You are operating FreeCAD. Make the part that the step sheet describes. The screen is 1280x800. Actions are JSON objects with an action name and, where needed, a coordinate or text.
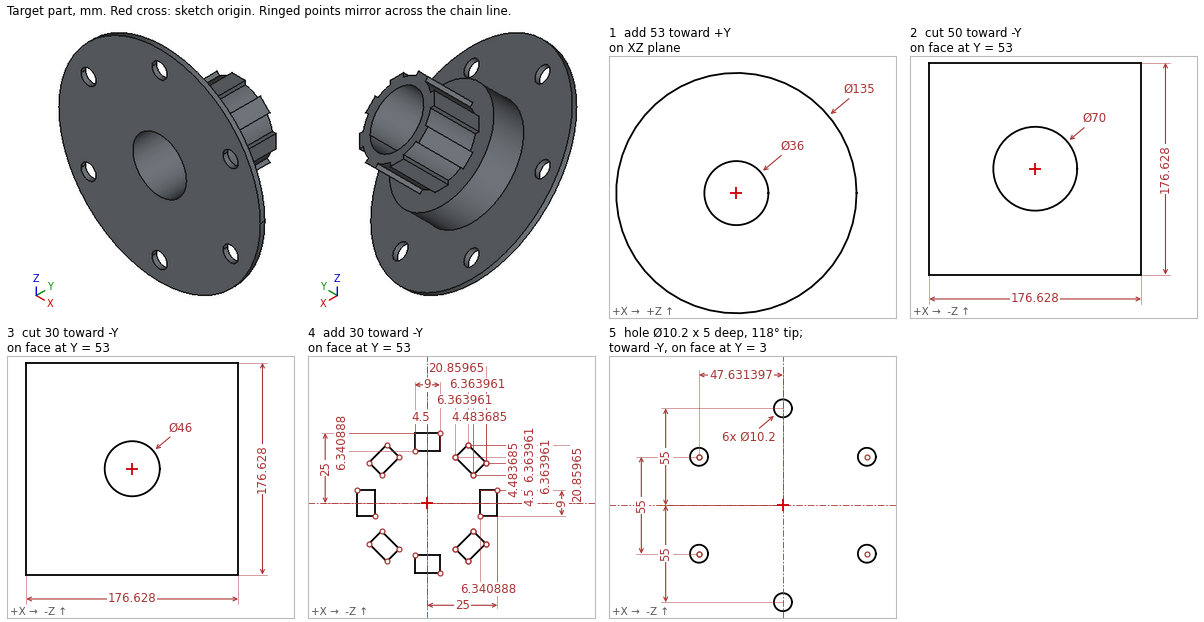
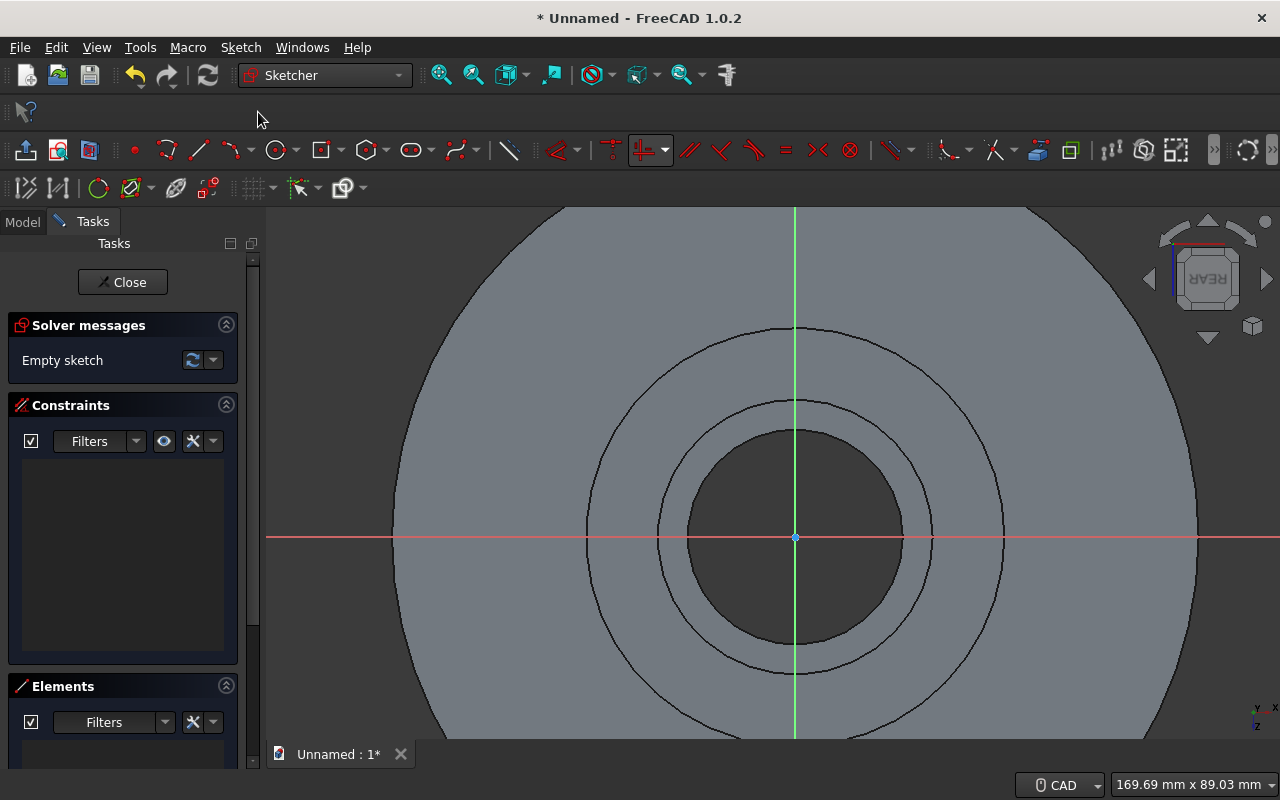
{"action": "scroll", "coordinate": [1115, 711], "scroll_direction": "up", "scroll_amount": 1}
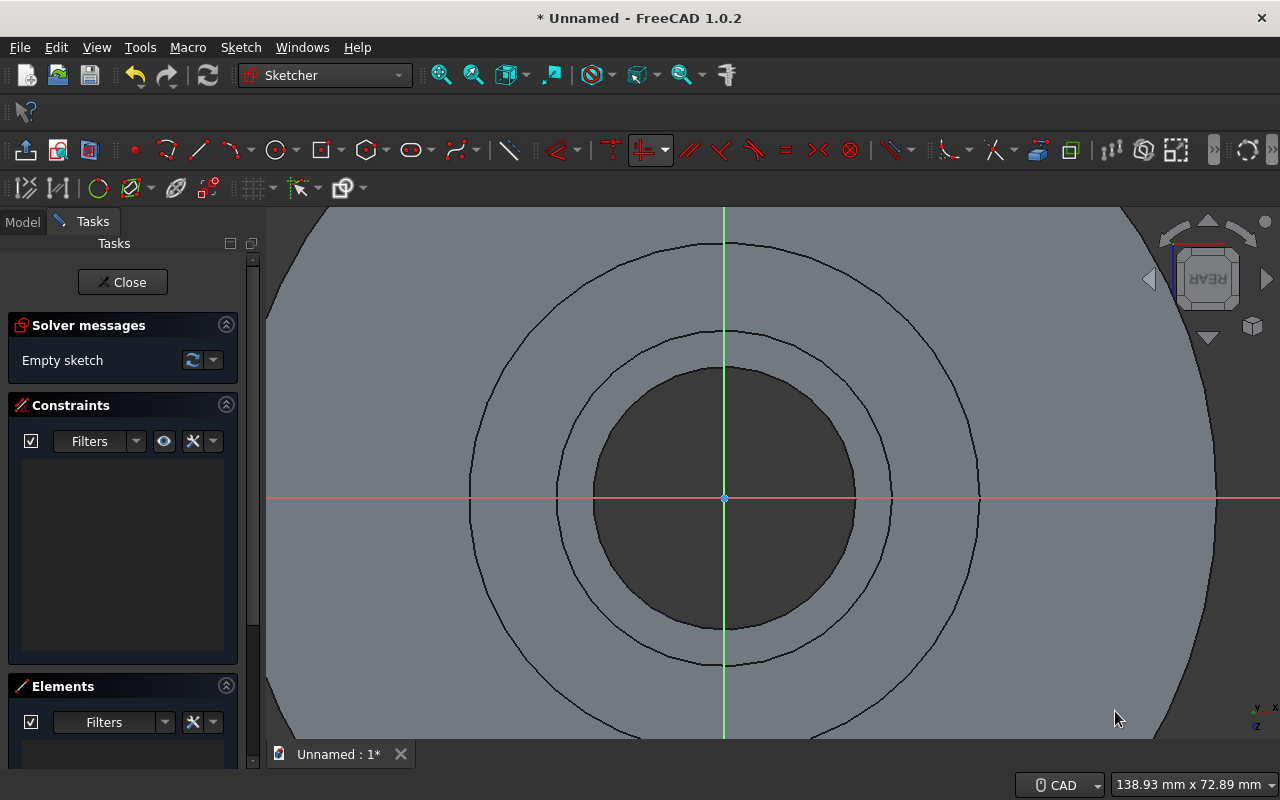
{"action": "left_click", "coordinate": [344, 150]}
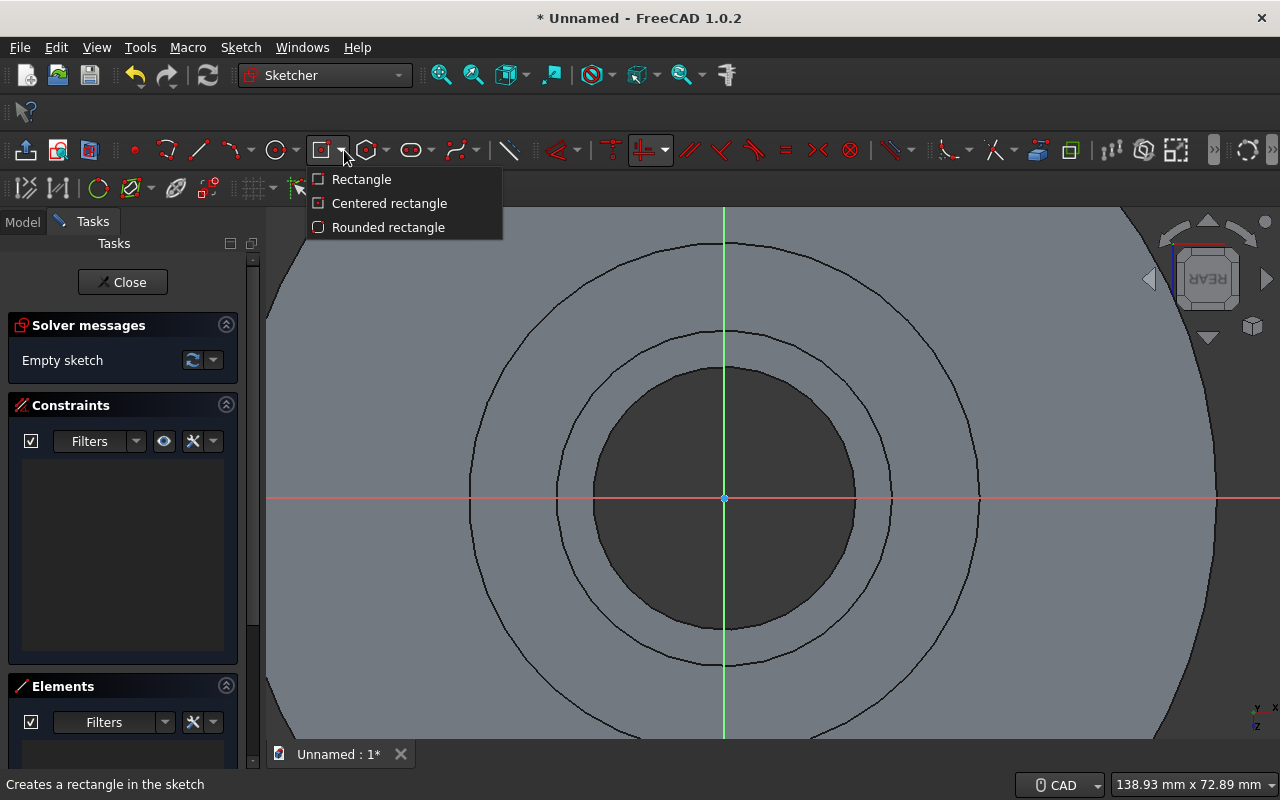
{"action": "left_click", "coordinate": [404, 179]}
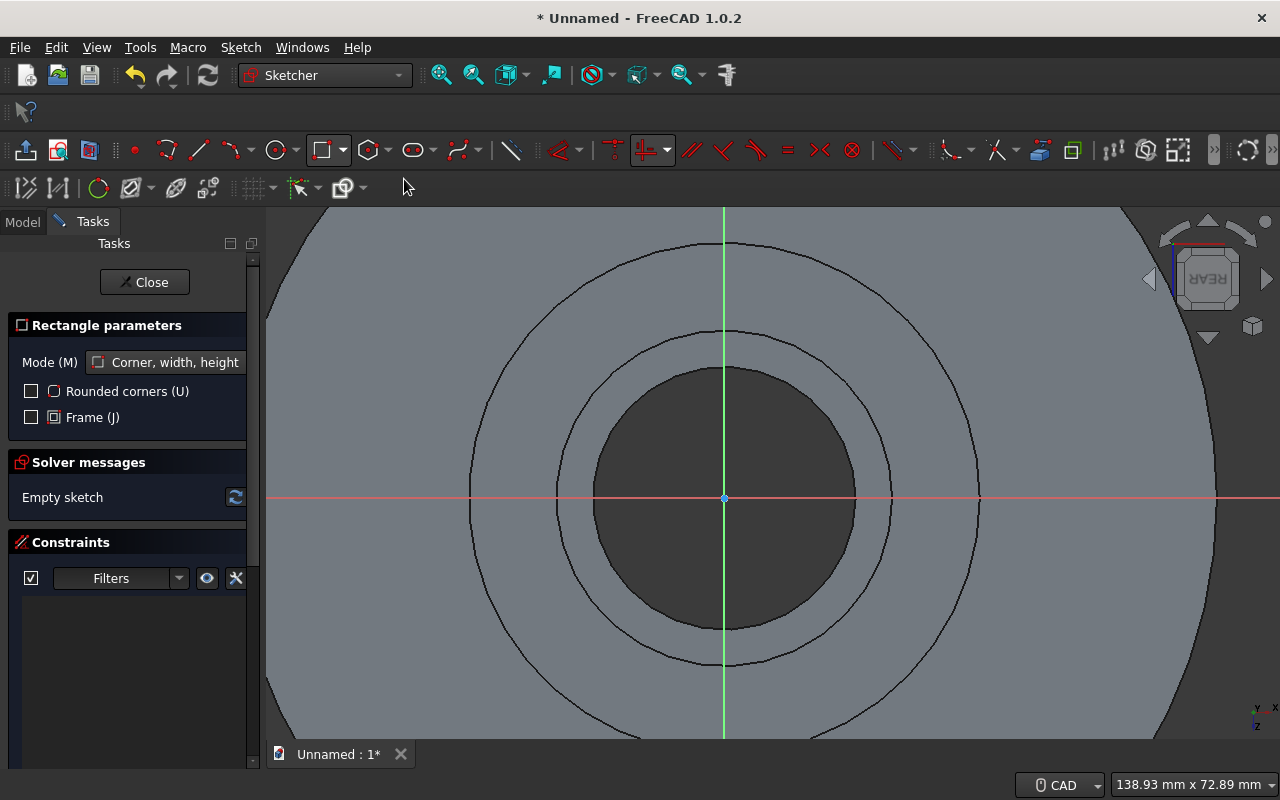
{"action": "left_click", "coordinate": [691, 316]}
{"action": "left_click", "coordinate": [757, 362]}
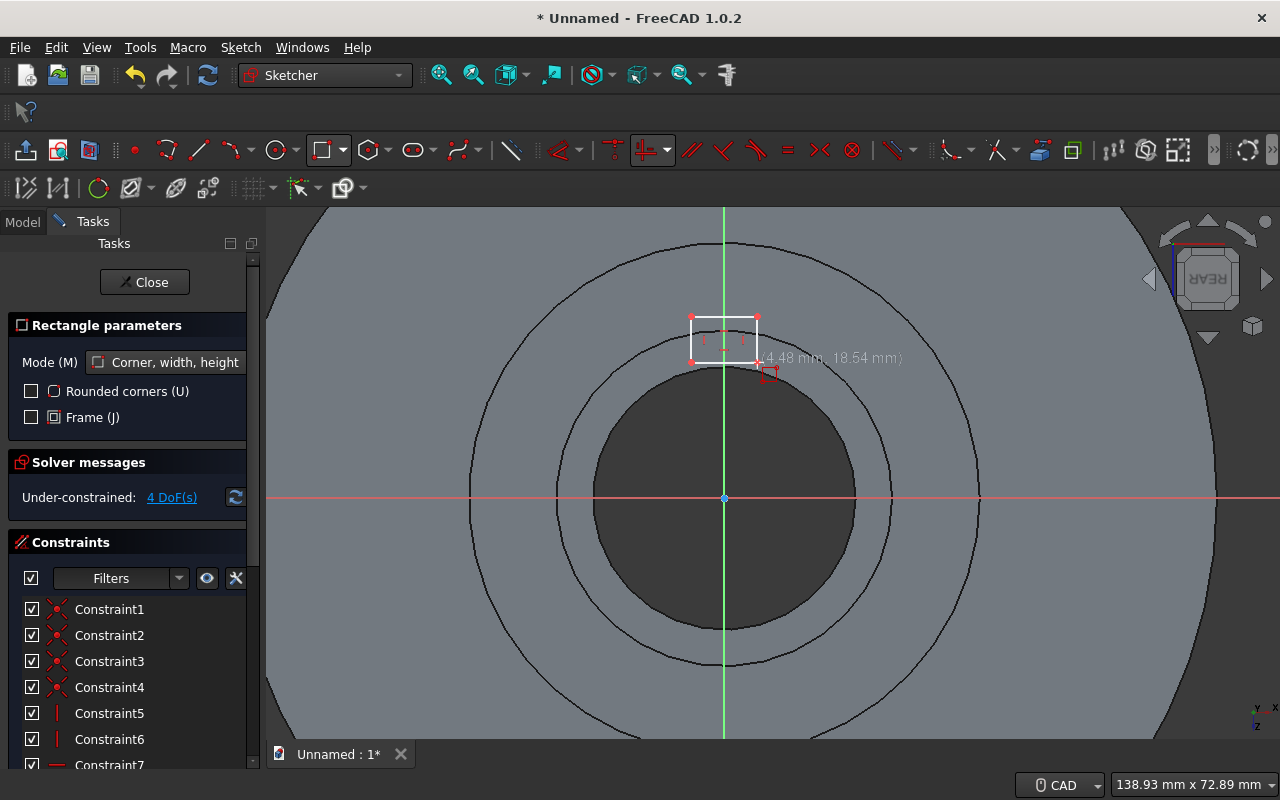
{"action": "left_click", "coordinate": [168, 150]}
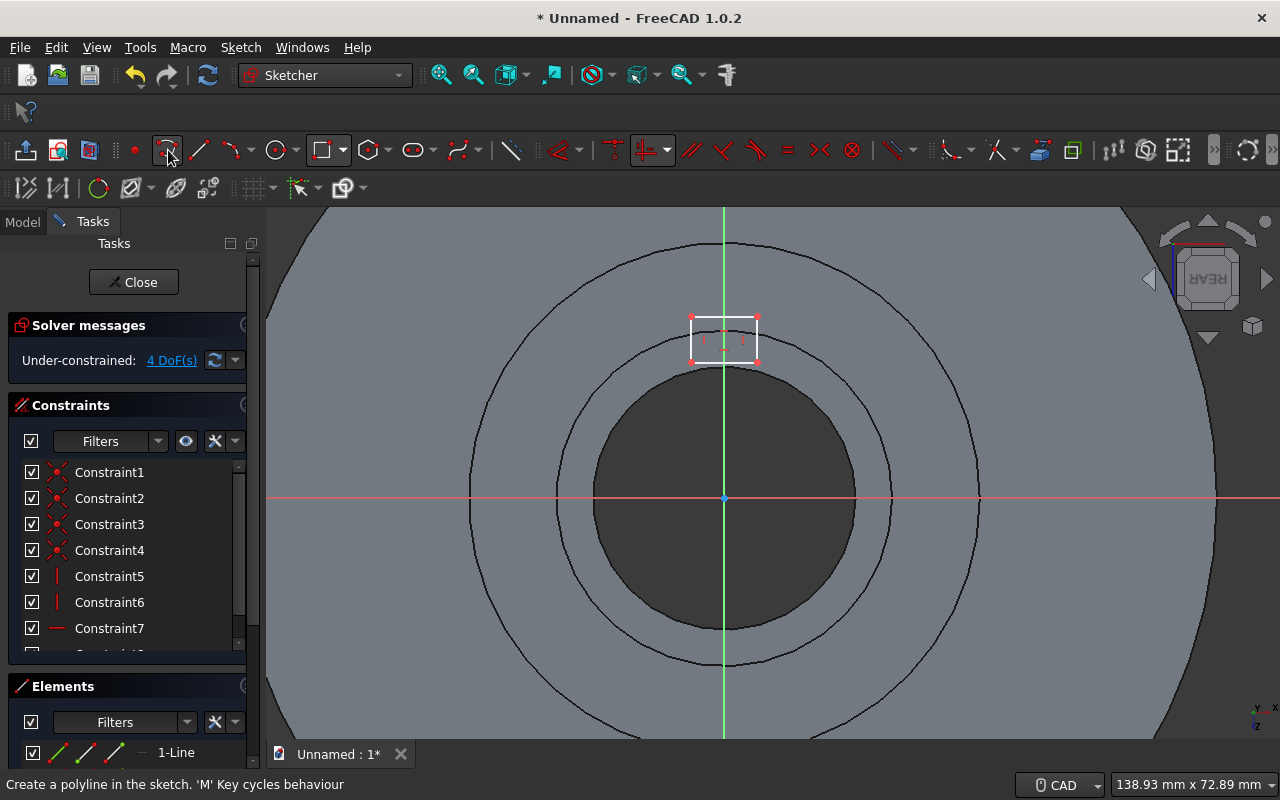
{"action": "left_click", "coordinate": [797, 379]}
{"action": "left_click", "coordinate": [844, 425]}
{"action": "left_click", "coordinate": [877, 393]}
{"action": "left_click", "coordinate": [830, 346]}
{"action": "left_click", "coordinate": [797, 380]}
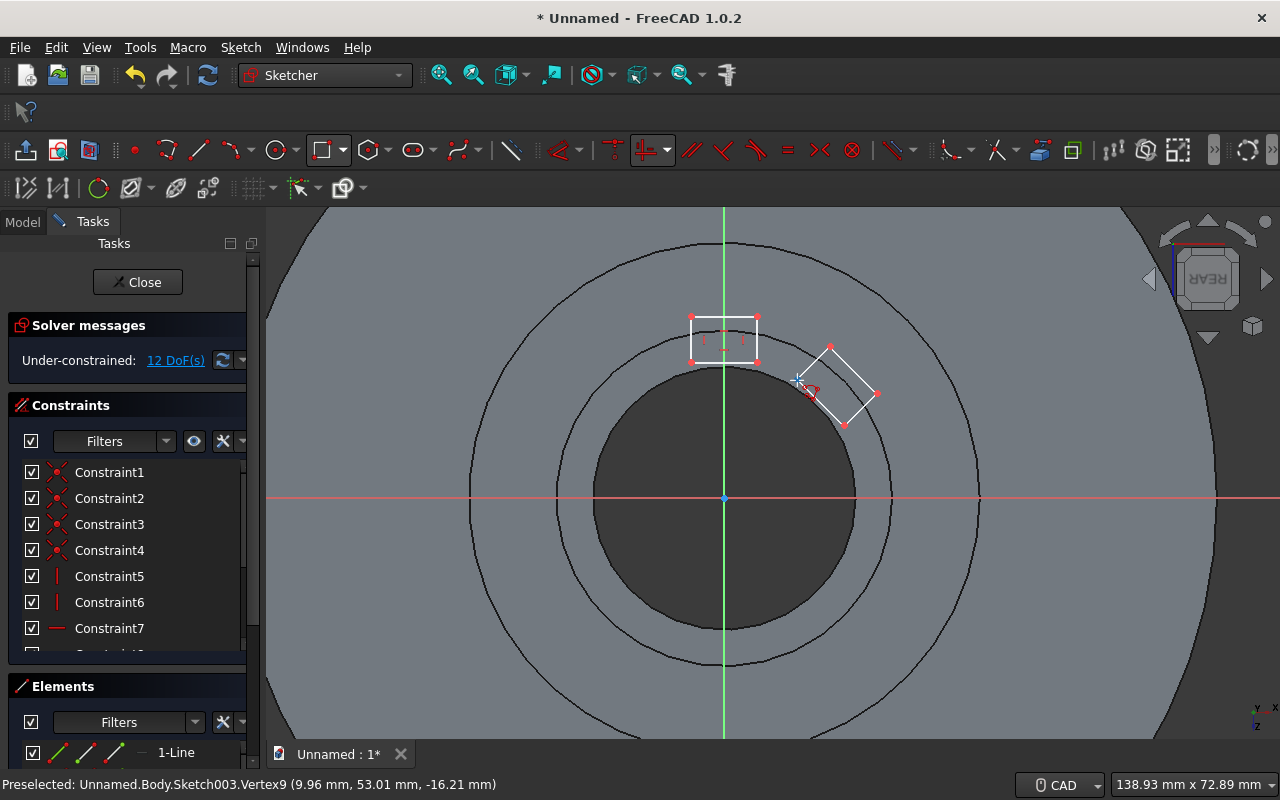
{"action": "left_click", "coordinate": [322, 150]}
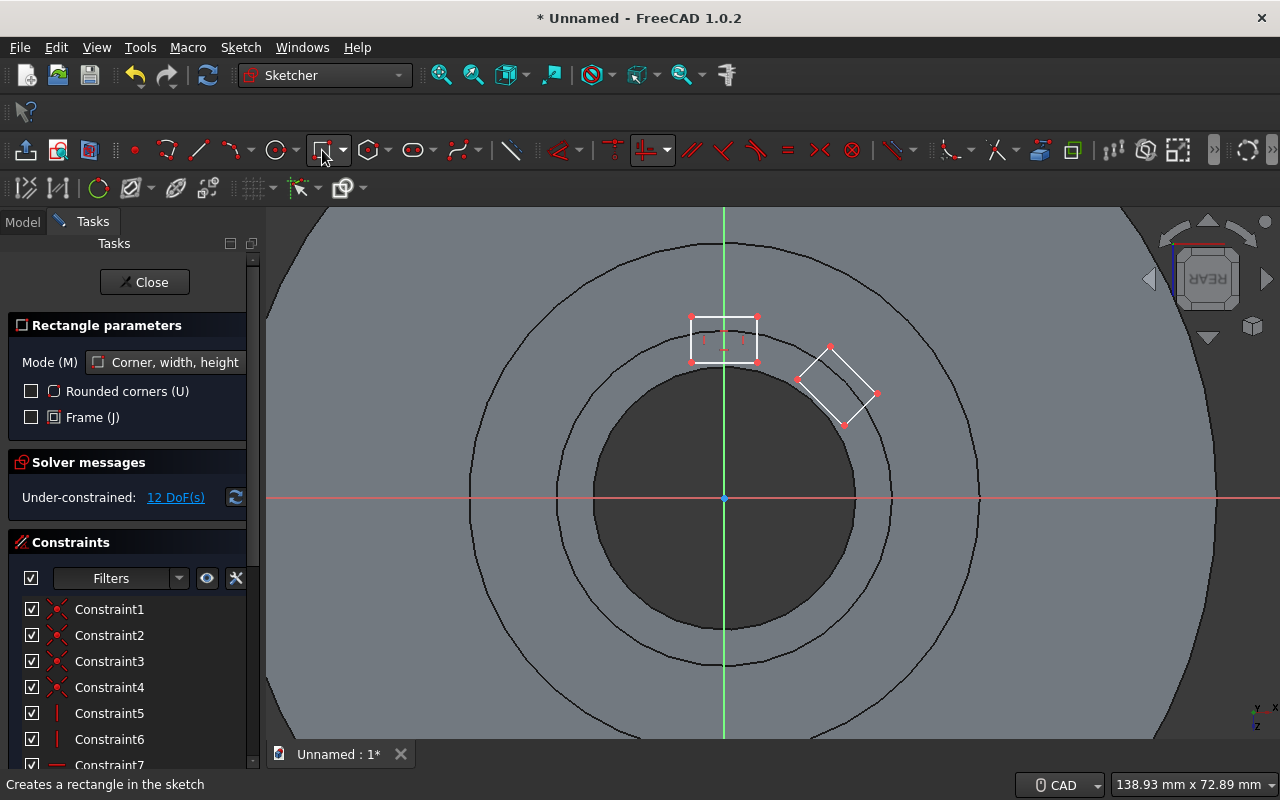
{"action": "left_click", "coordinate": [861, 465]}
{"action": "left_click", "coordinate": [907, 531]}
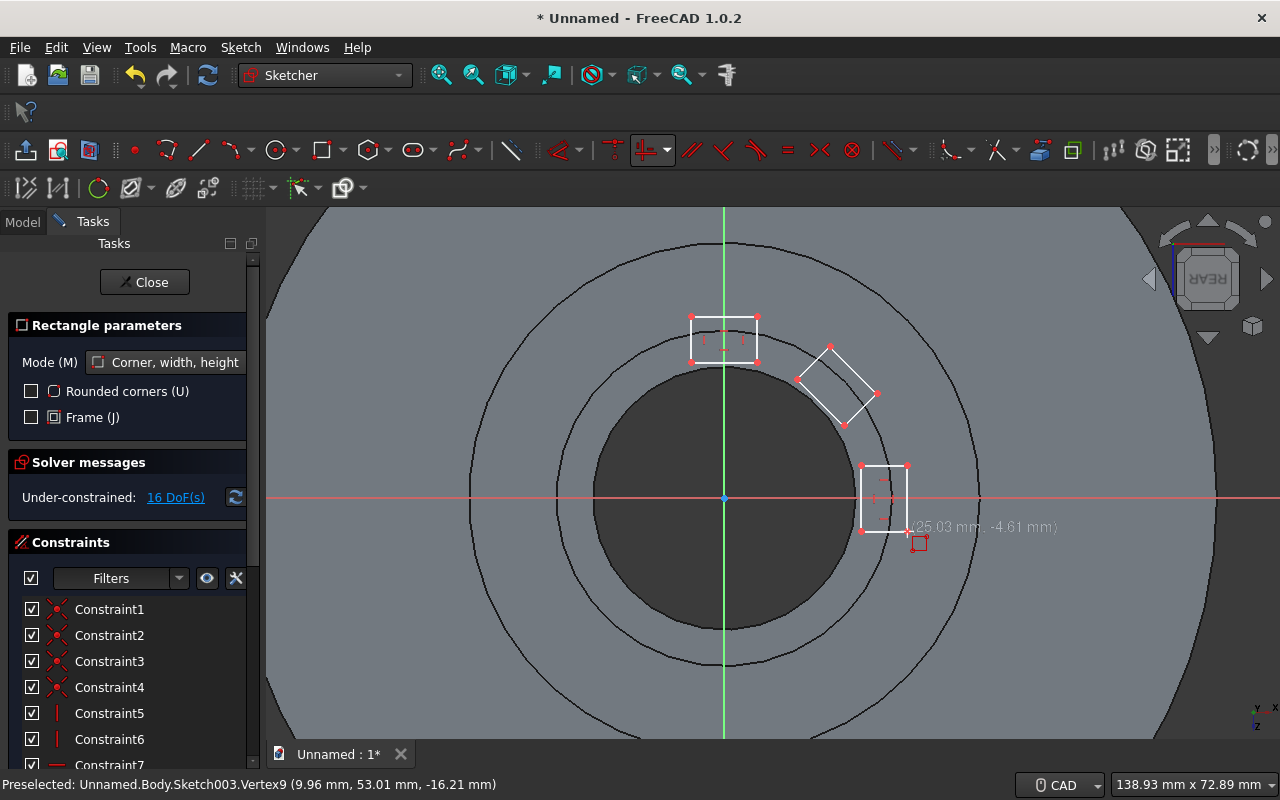
{"action": "left_click", "coordinate": [168, 150]}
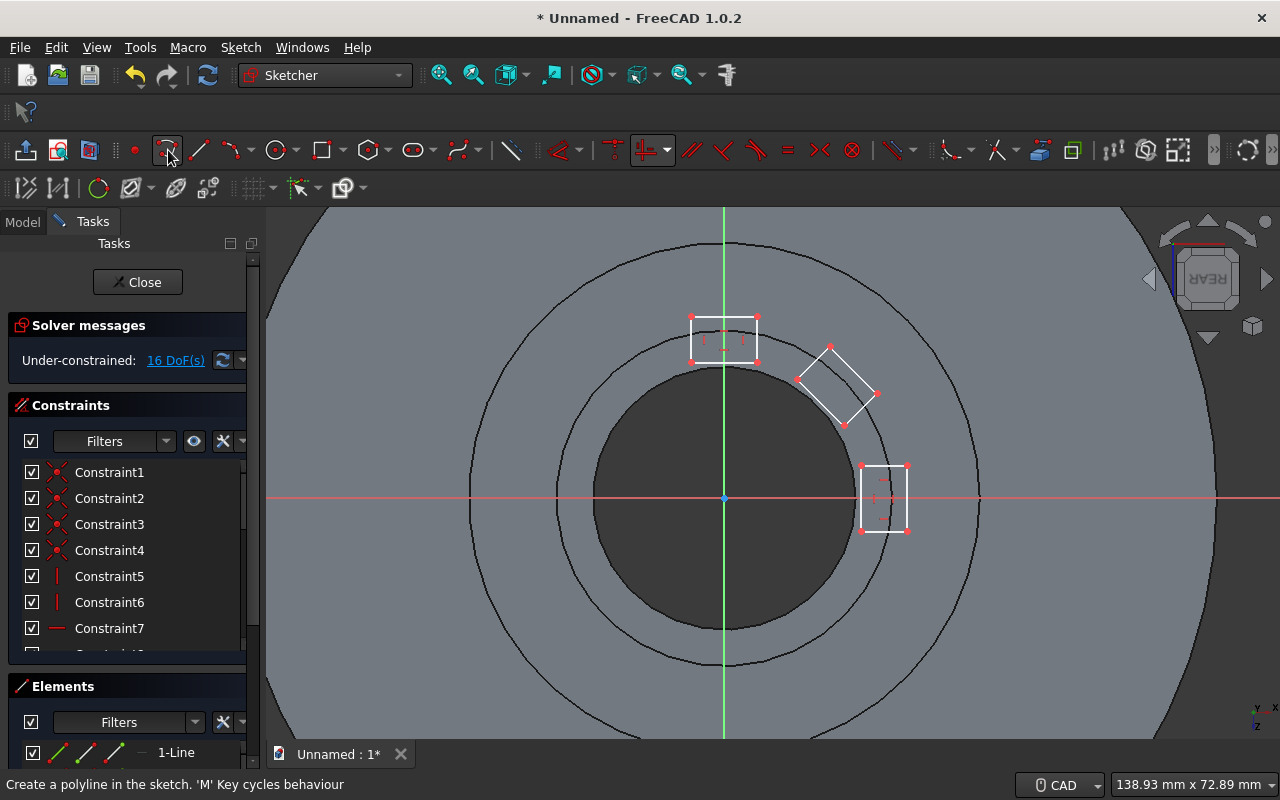
{"action": "left_click", "coordinate": [844, 571]}
{"action": "left_click", "coordinate": [797, 618]}
{"action": "left_click", "coordinate": [830, 651]}
{"action": "left_click", "coordinate": [877, 604]}
{"action": "left_click", "coordinate": [844, 572]}